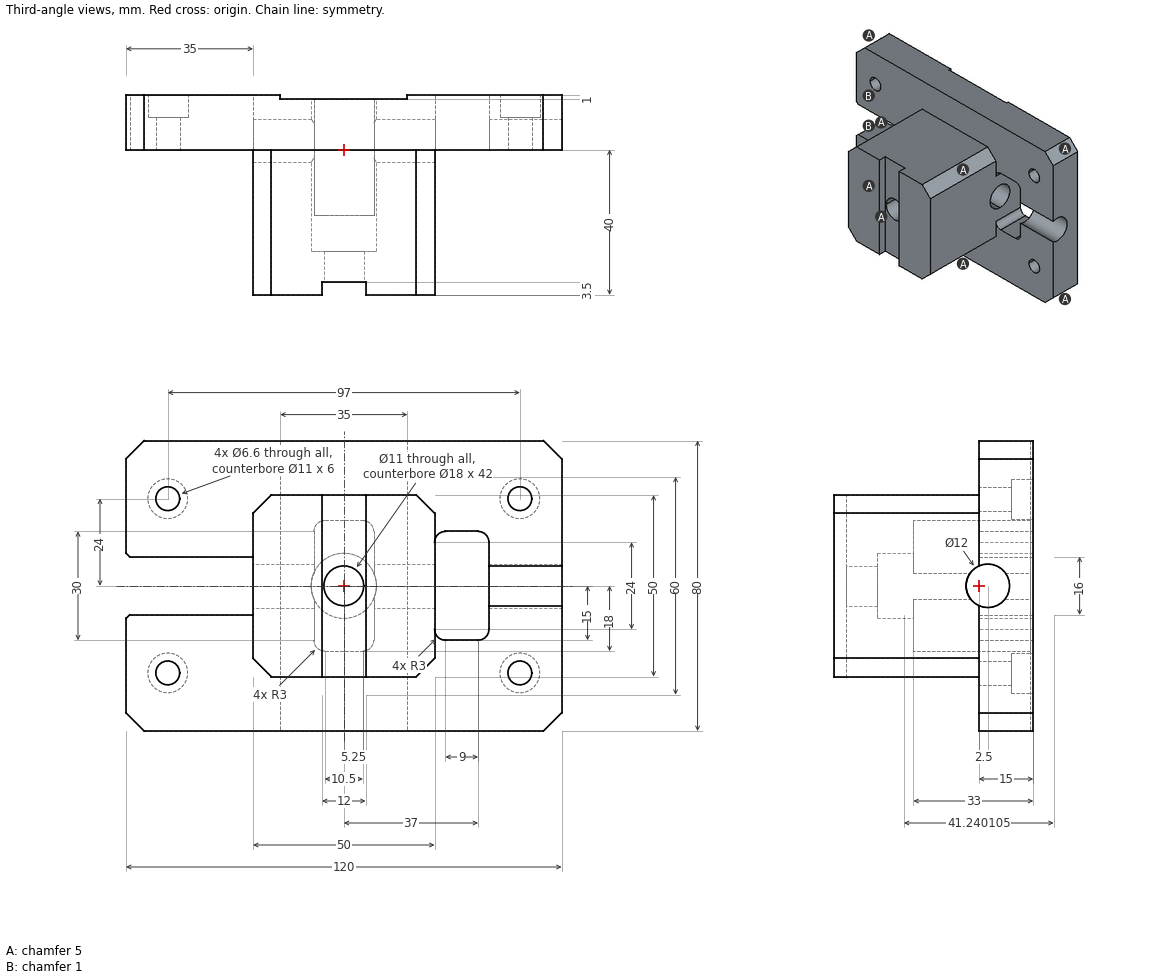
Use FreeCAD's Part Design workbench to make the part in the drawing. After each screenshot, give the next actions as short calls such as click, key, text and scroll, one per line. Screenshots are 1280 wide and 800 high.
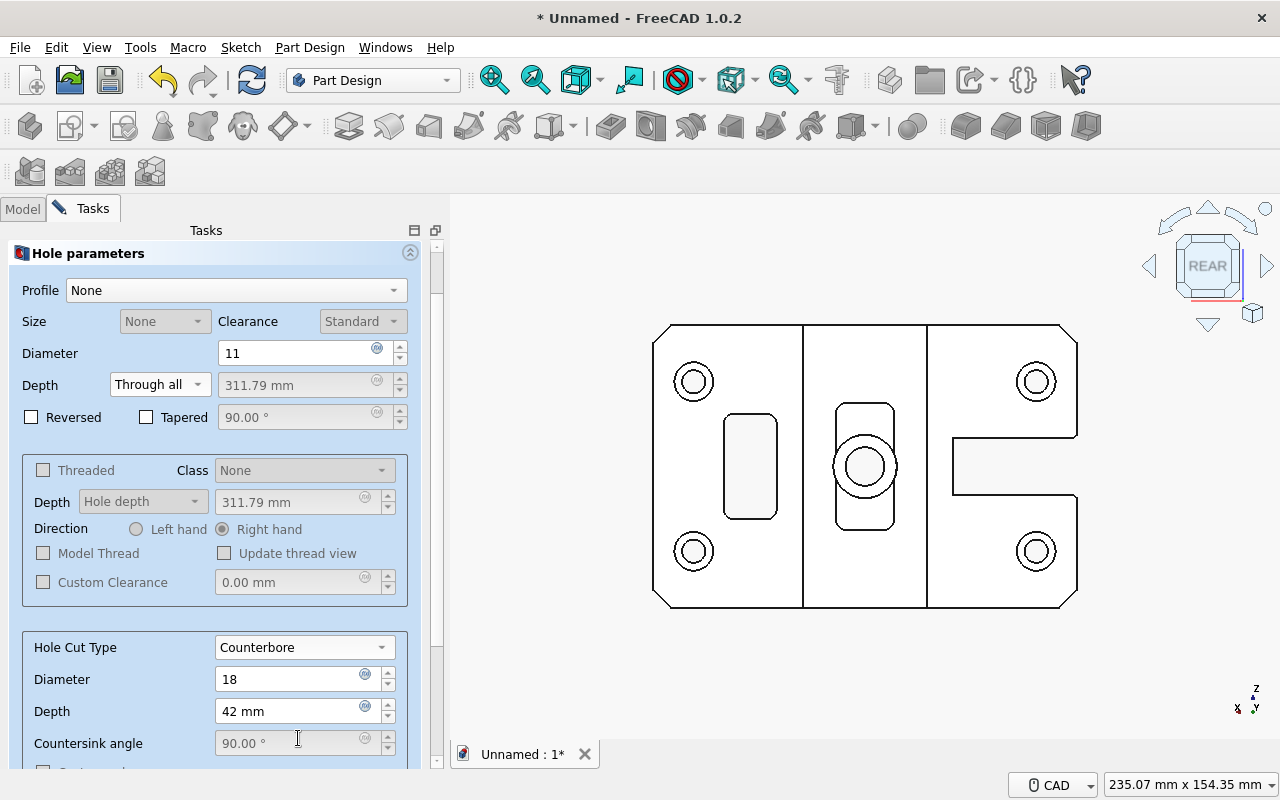
scroll(437, 504, up, 2)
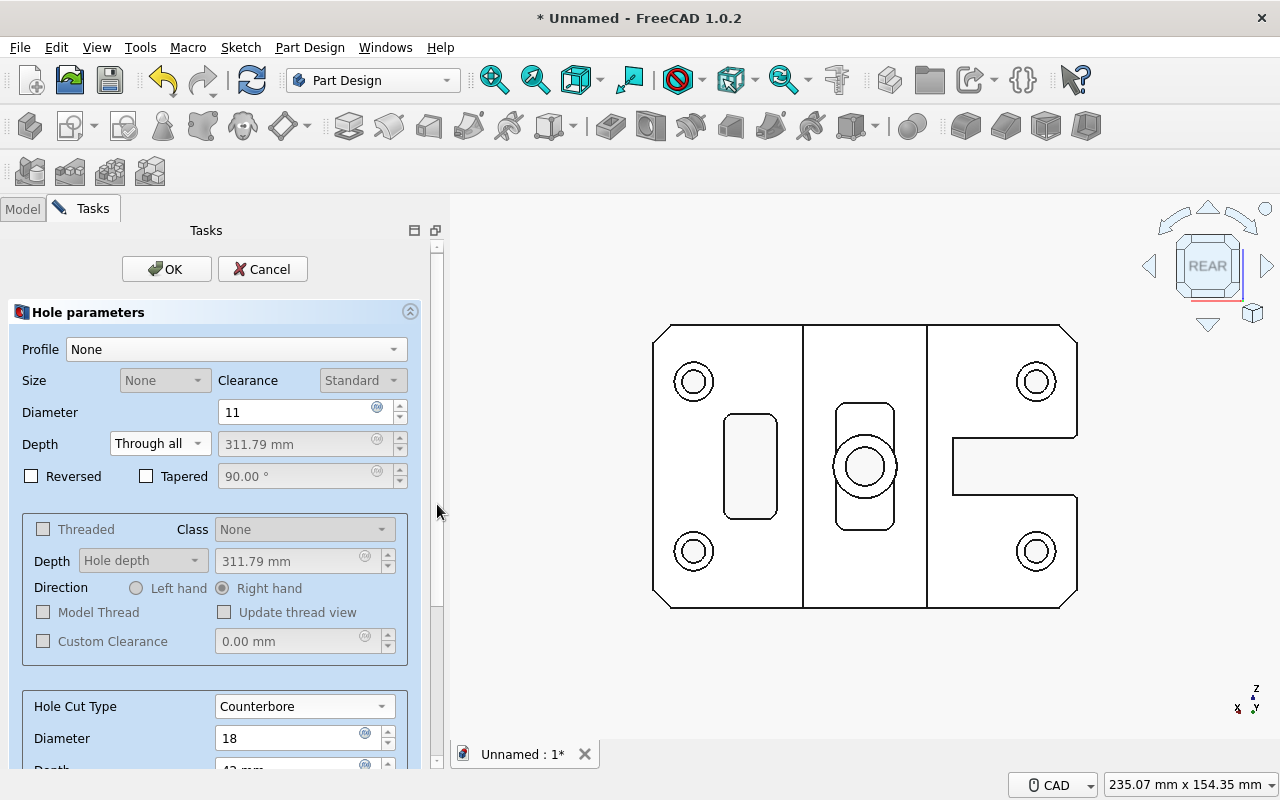
click(167, 269)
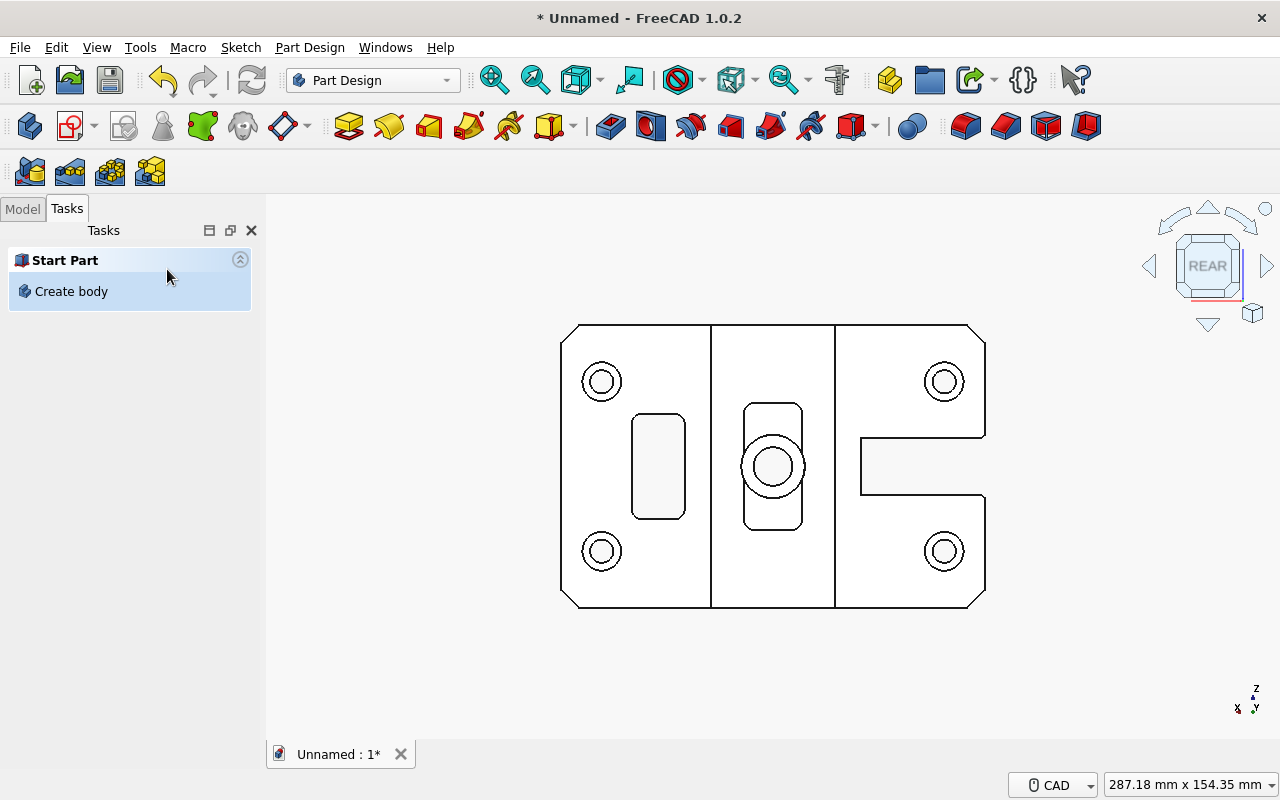
key(0)